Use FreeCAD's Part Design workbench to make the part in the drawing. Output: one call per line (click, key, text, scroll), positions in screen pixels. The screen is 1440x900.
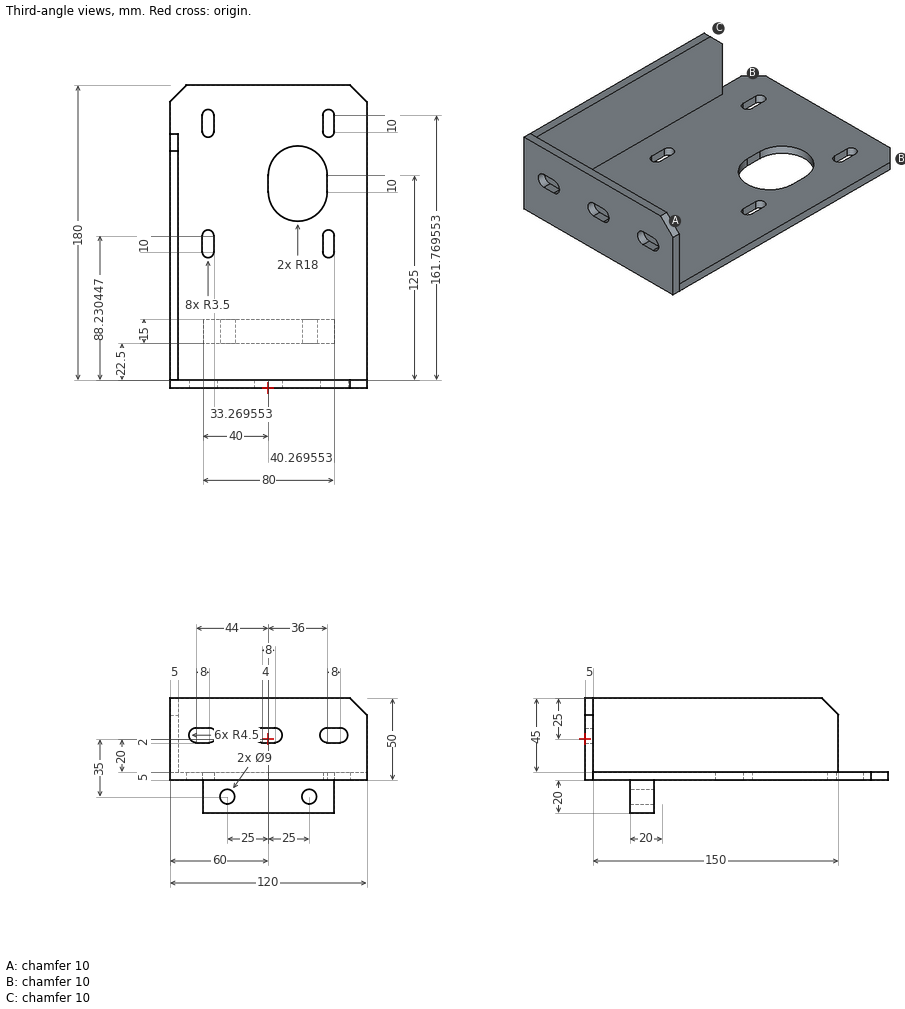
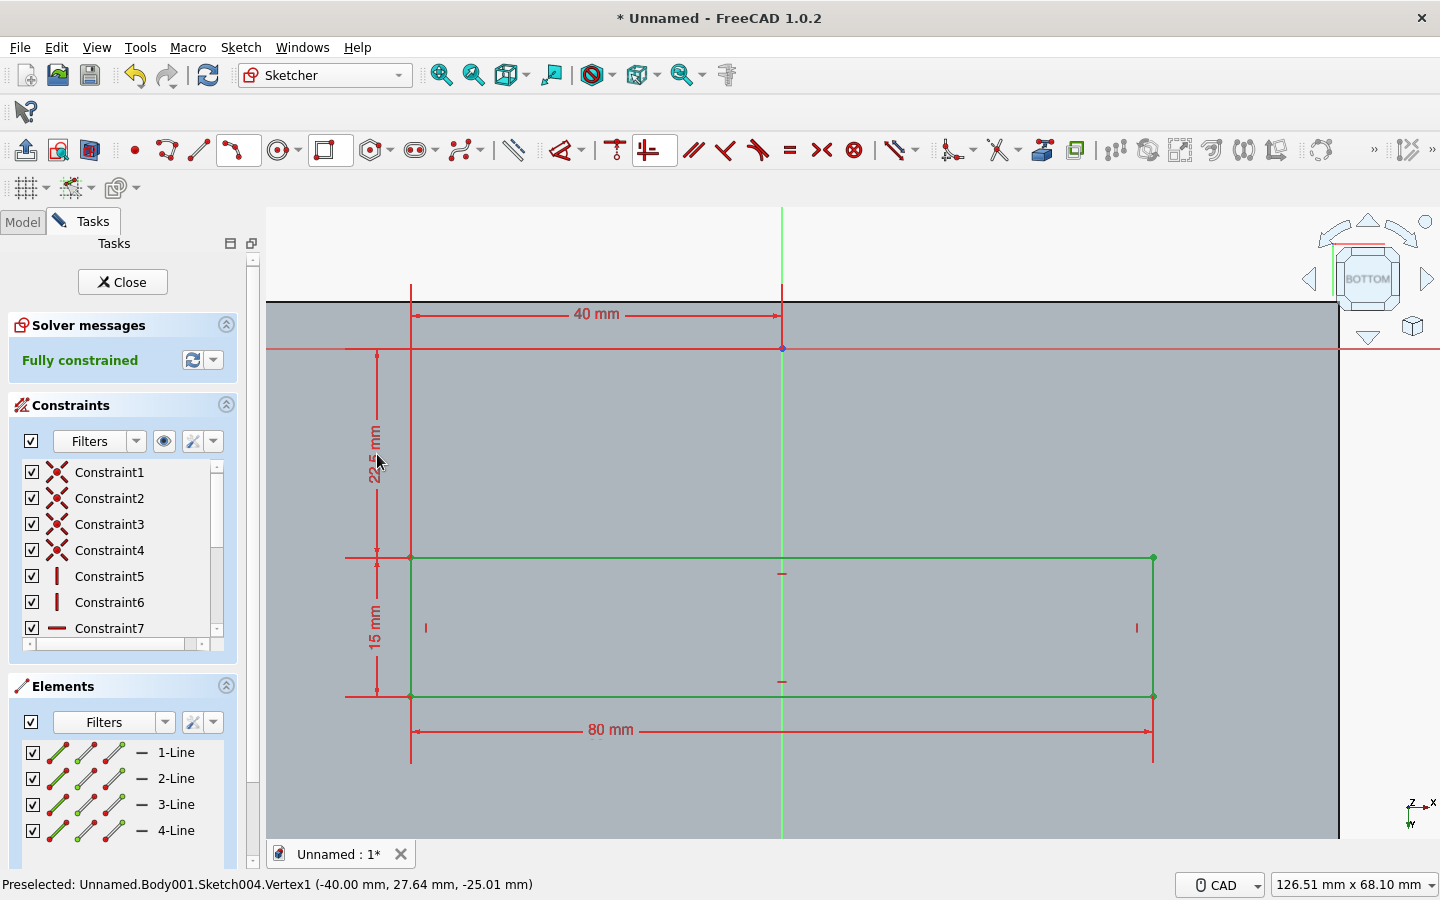
click(123, 282)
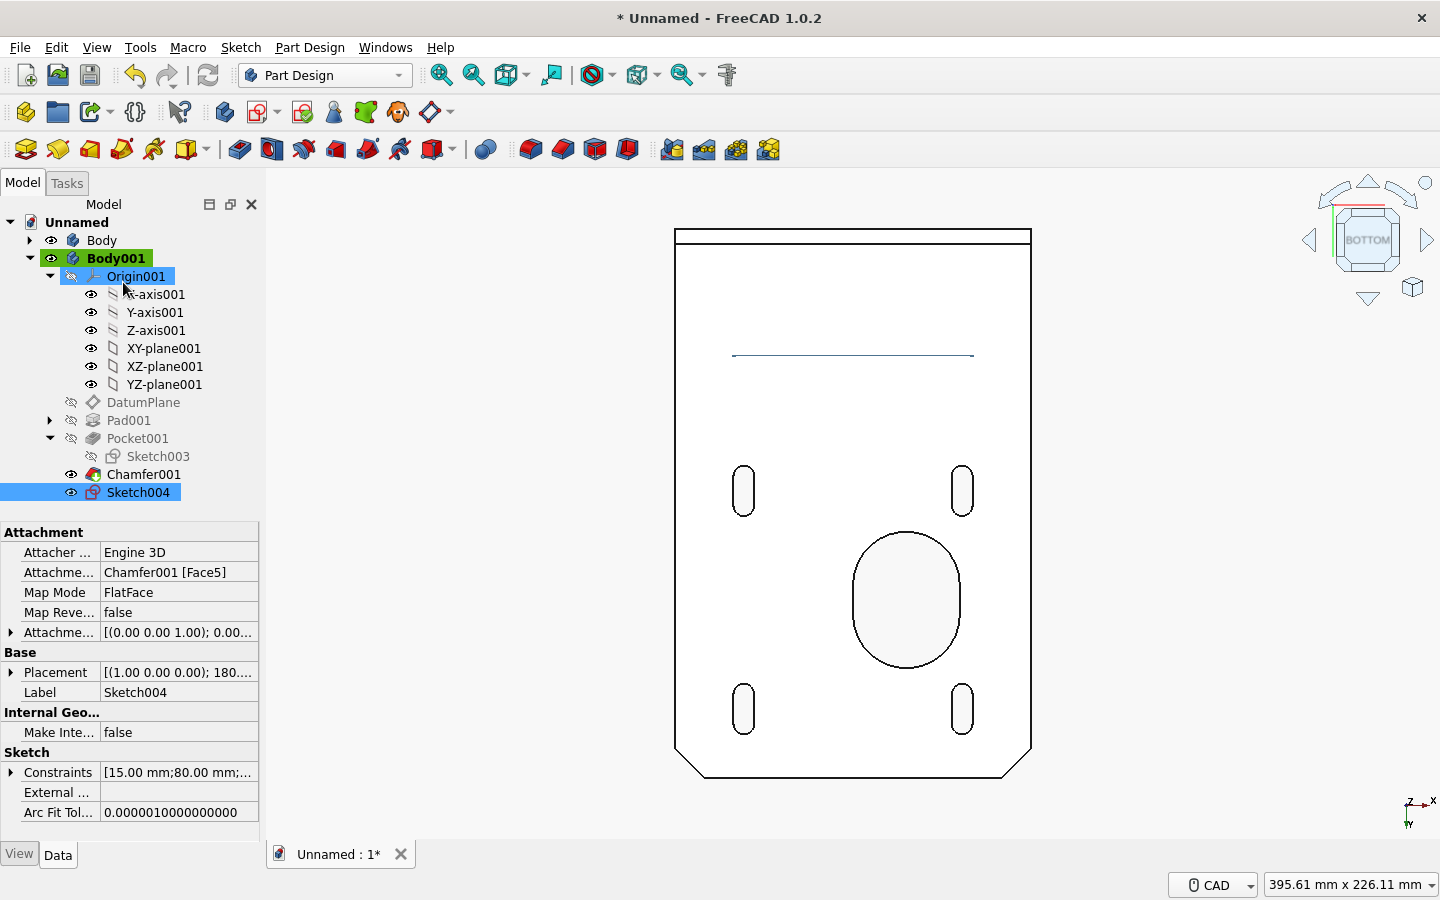
click(26, 150)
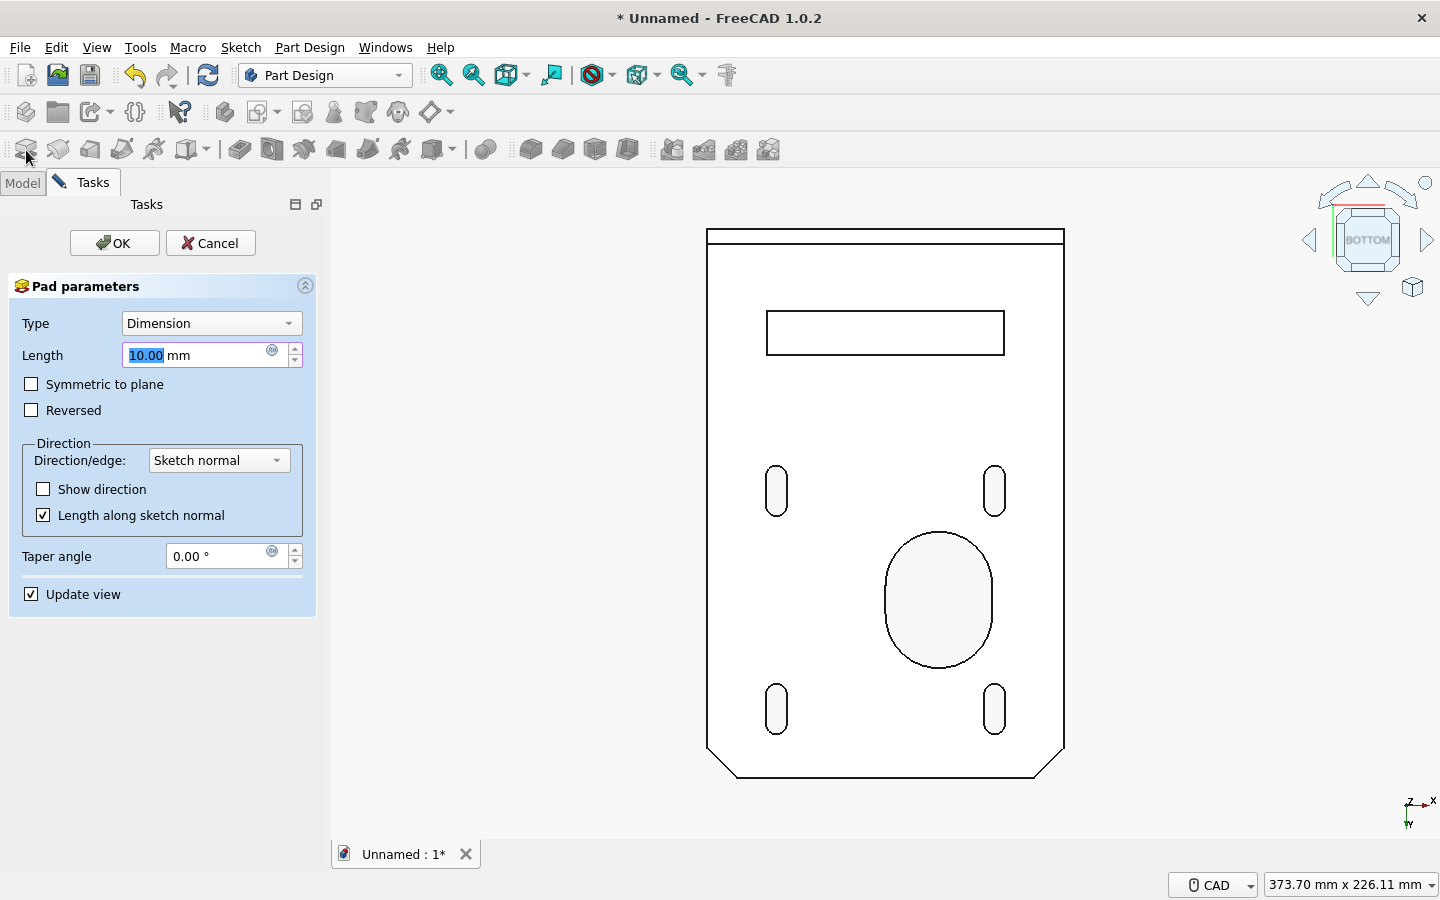
text(20)
key(Tab)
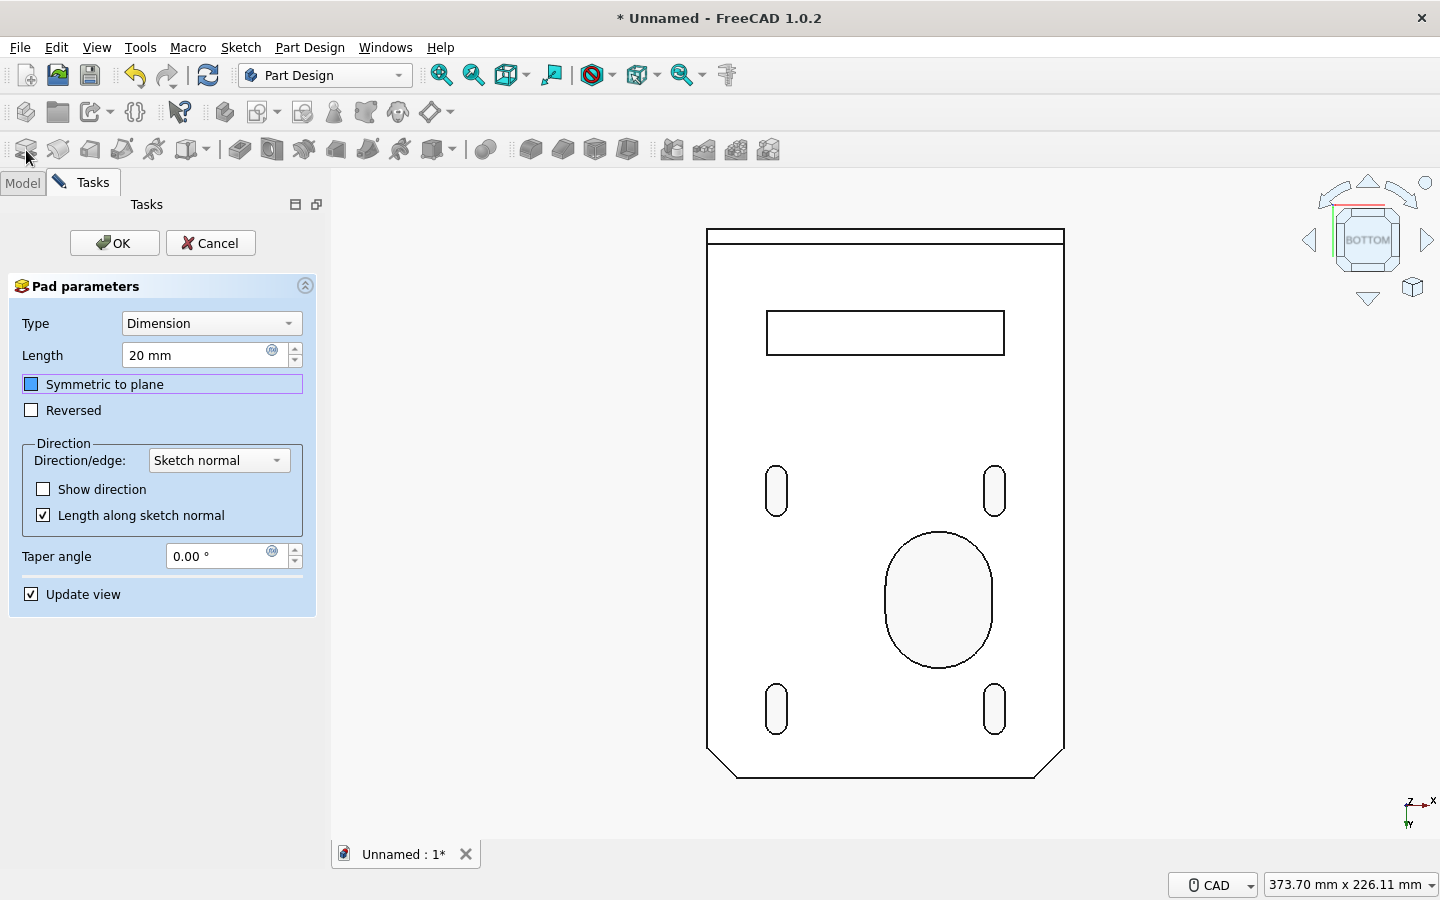
click(115, 243)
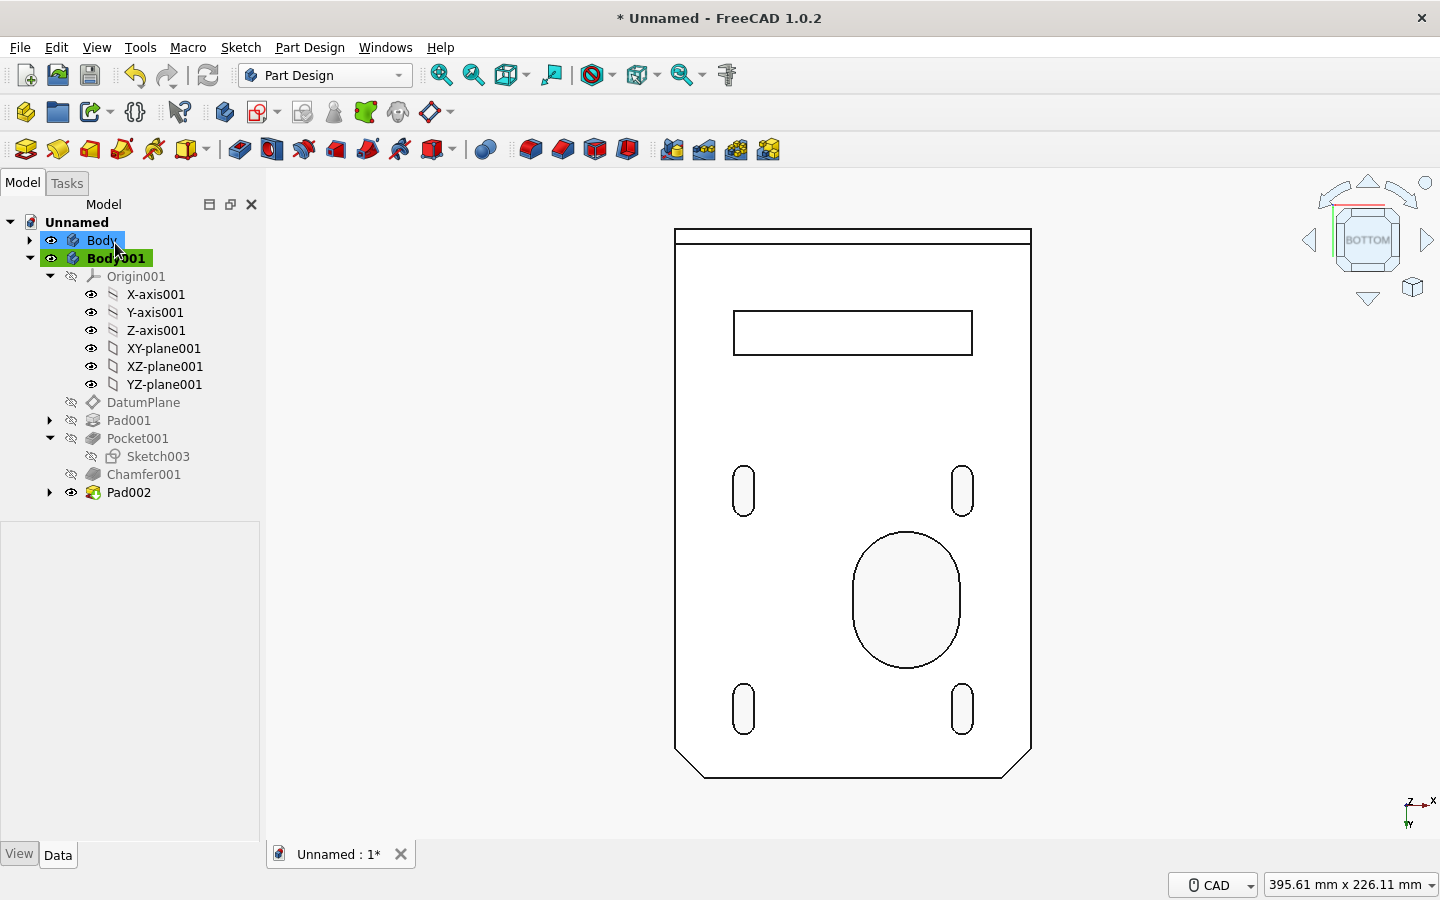
key(0)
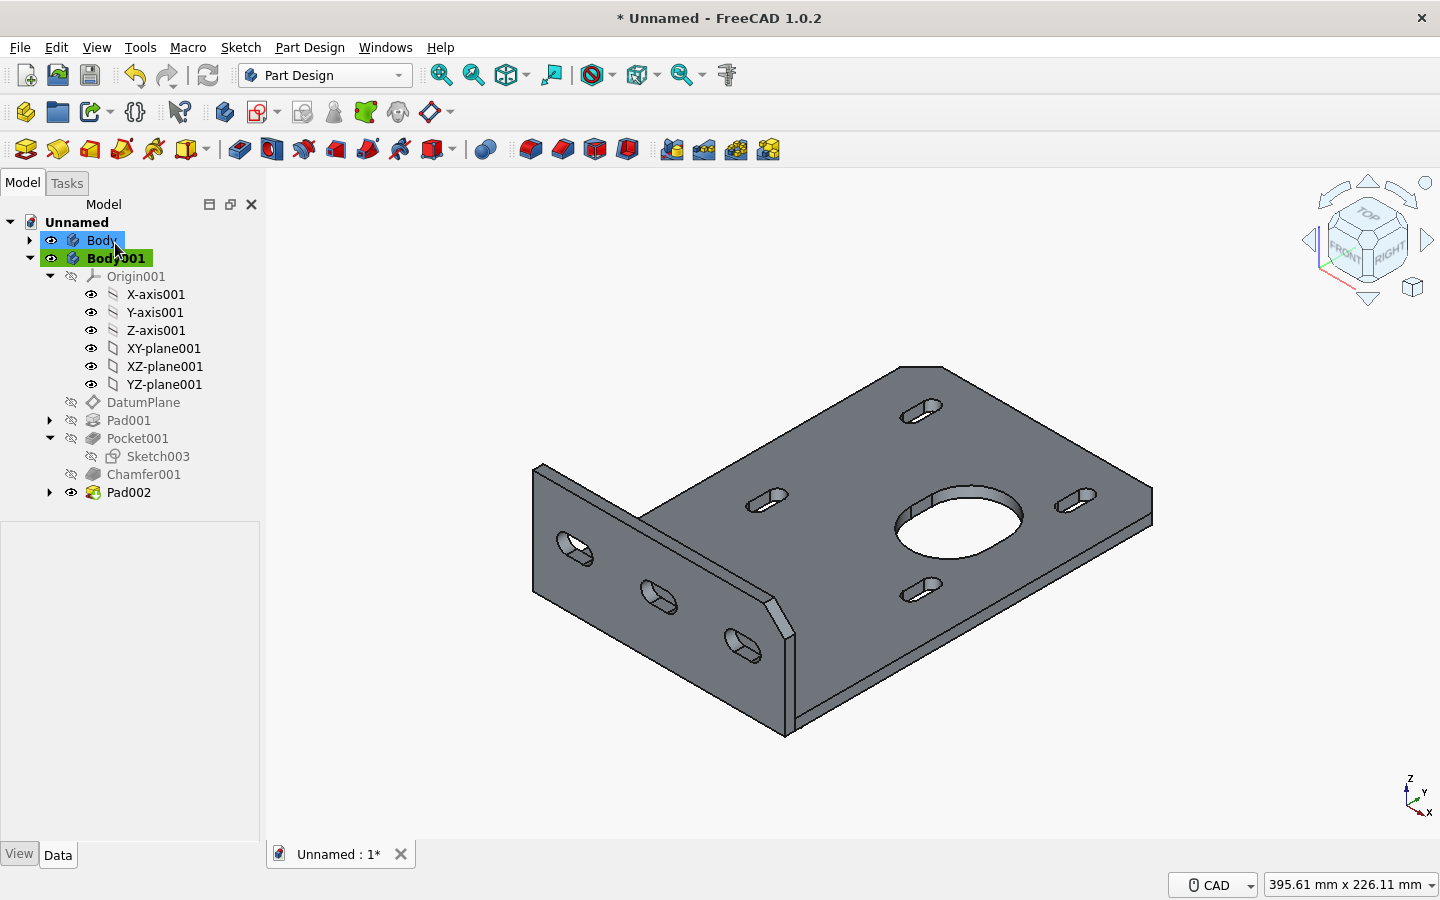
key(1)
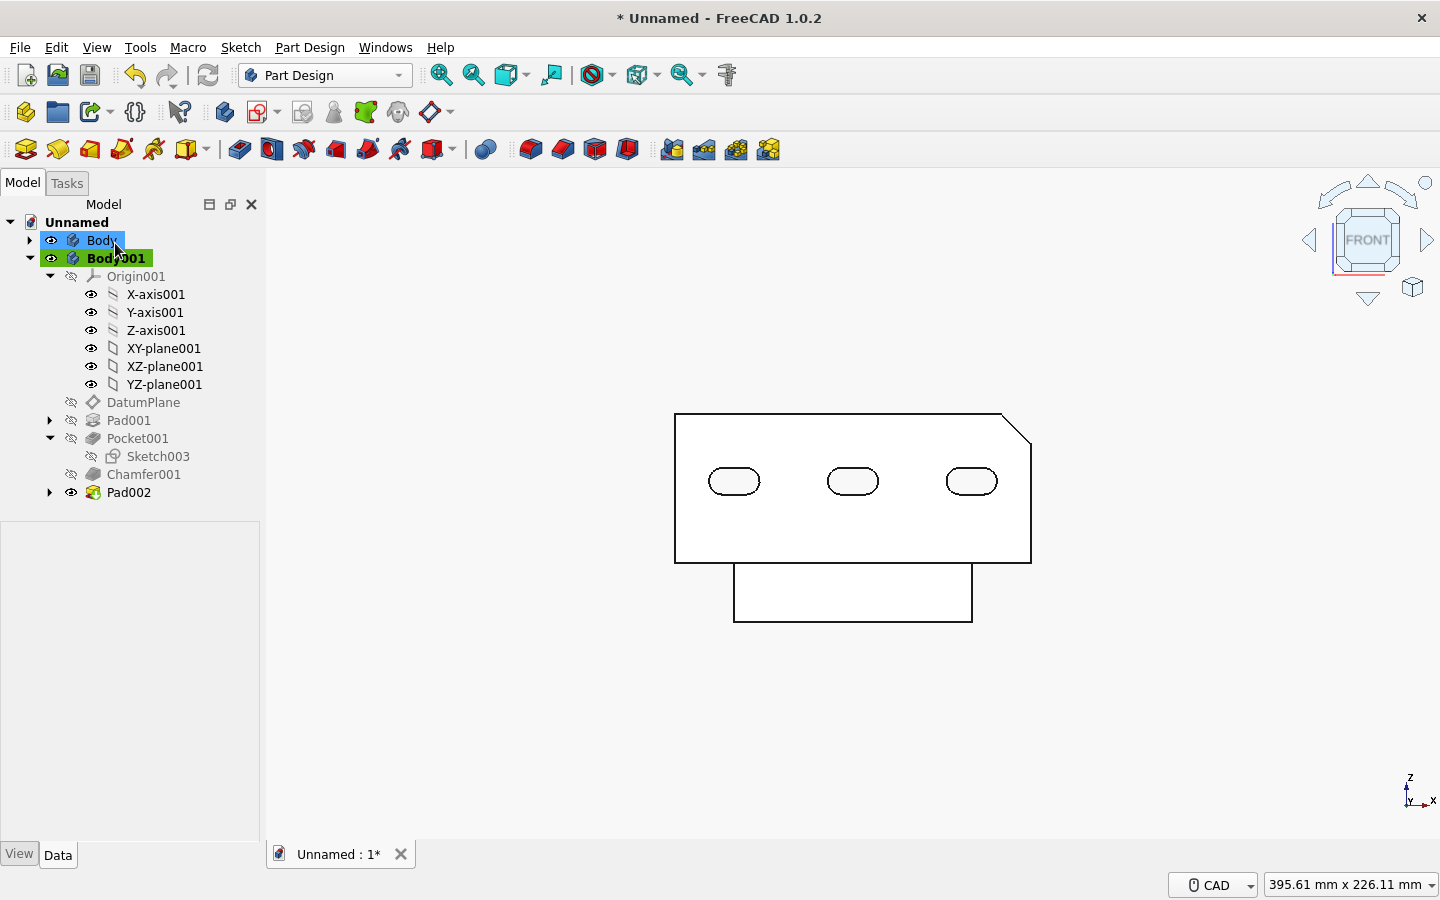
key(v)
key(f)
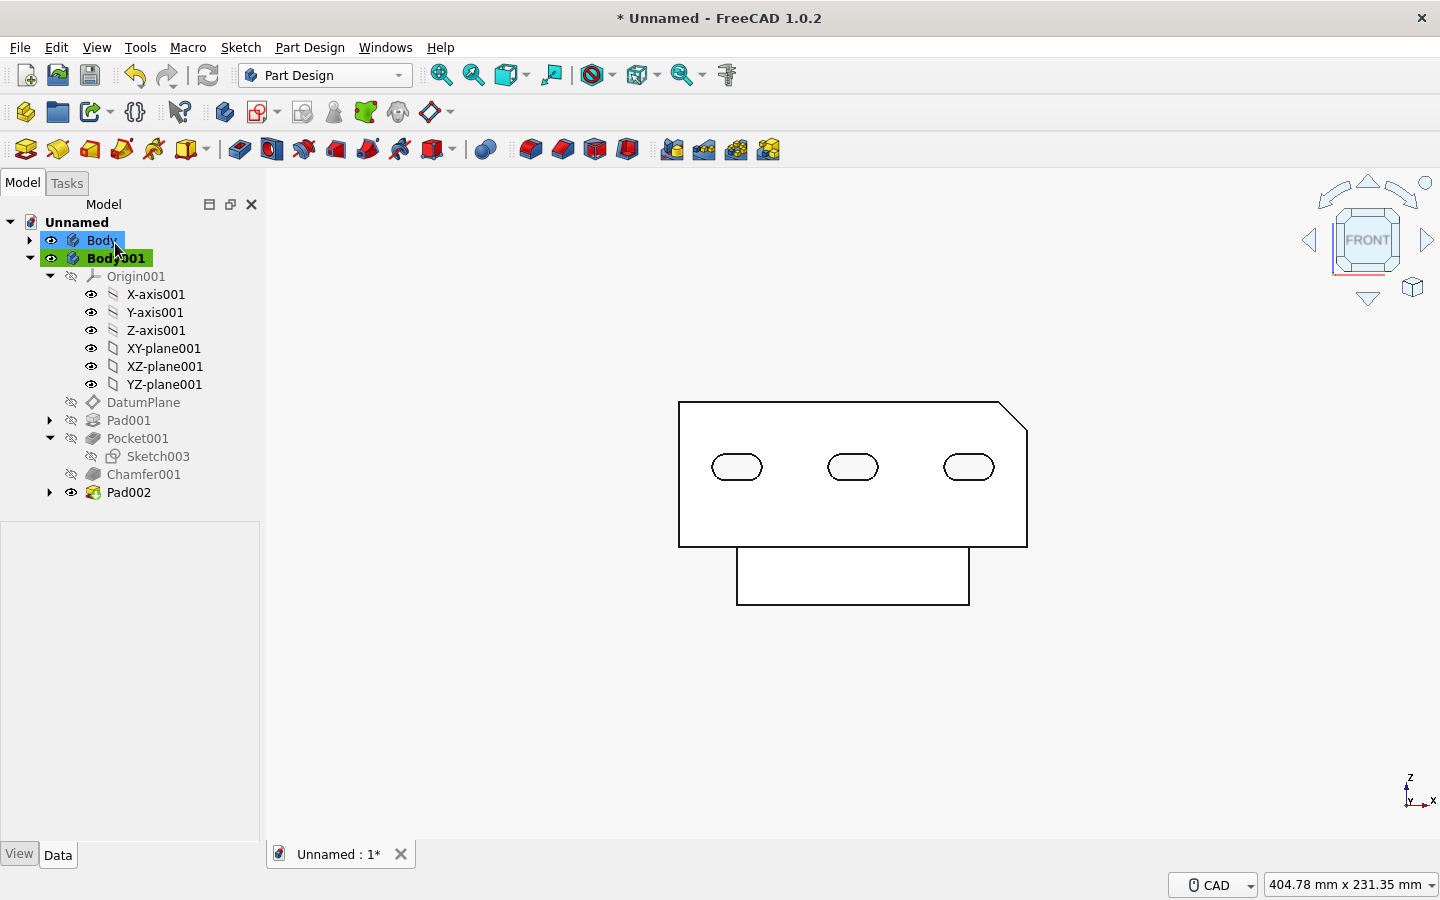
click(919, 575)